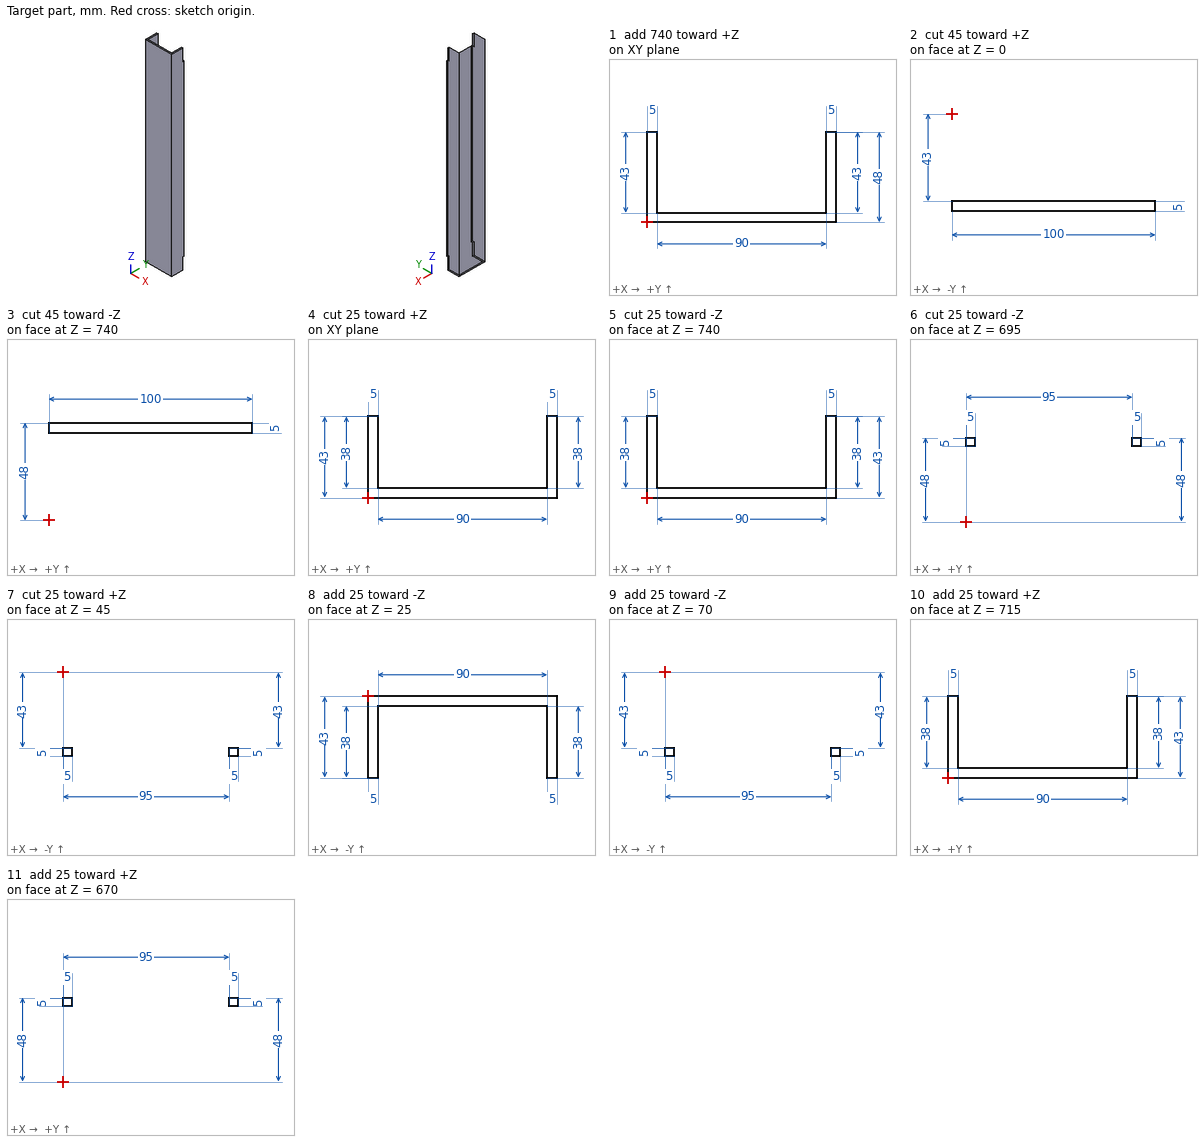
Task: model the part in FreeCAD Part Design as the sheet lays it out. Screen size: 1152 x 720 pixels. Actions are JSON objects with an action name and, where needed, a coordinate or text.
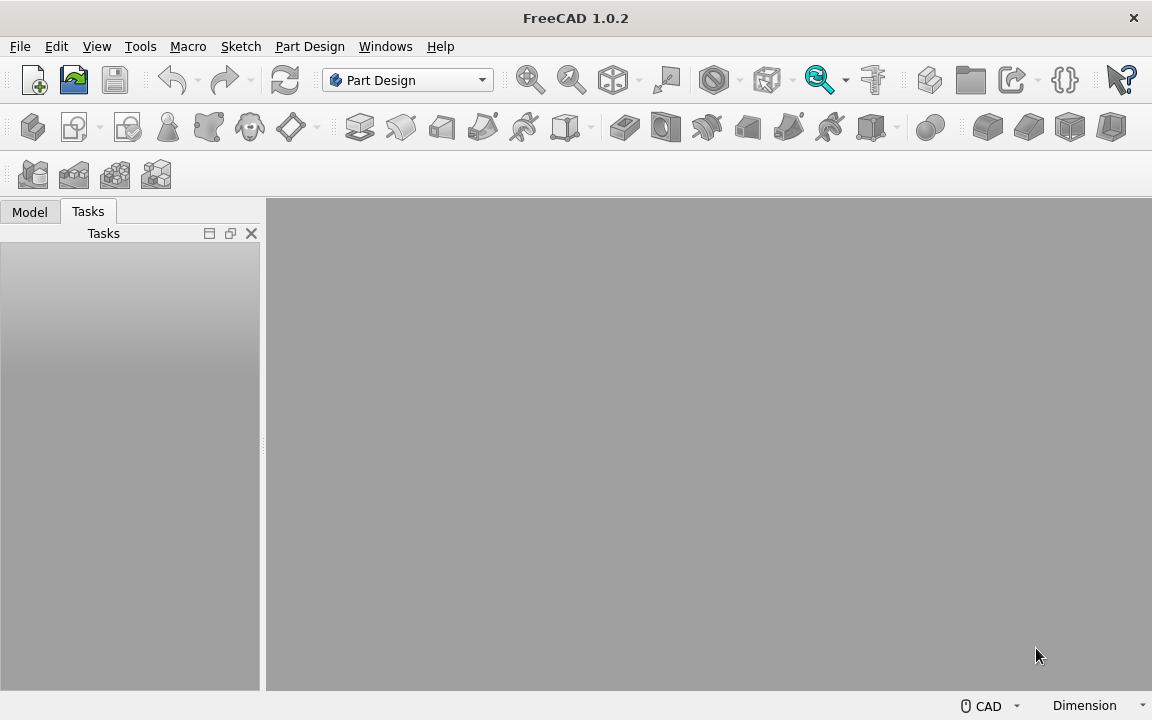
{"action": "left_click", "coordinate": [33, 80]}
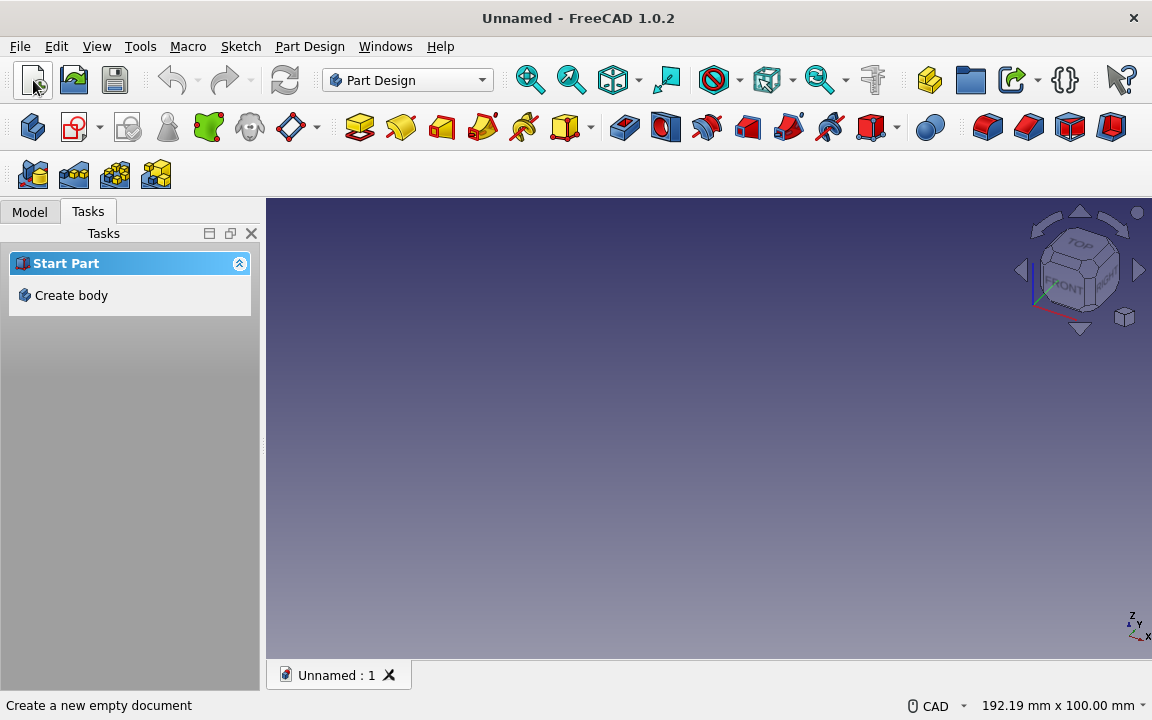
{"action": "left_click", "coordinate": [74, 128]}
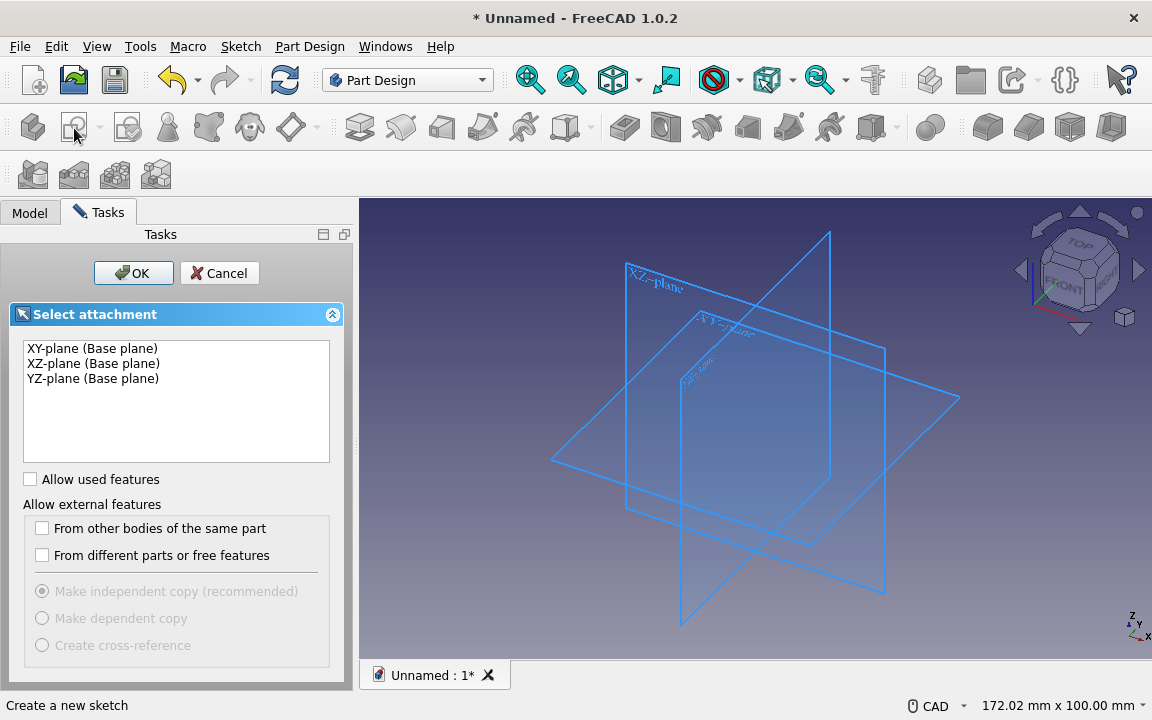
{"action": "left_click", "coordinate": [84, 348]}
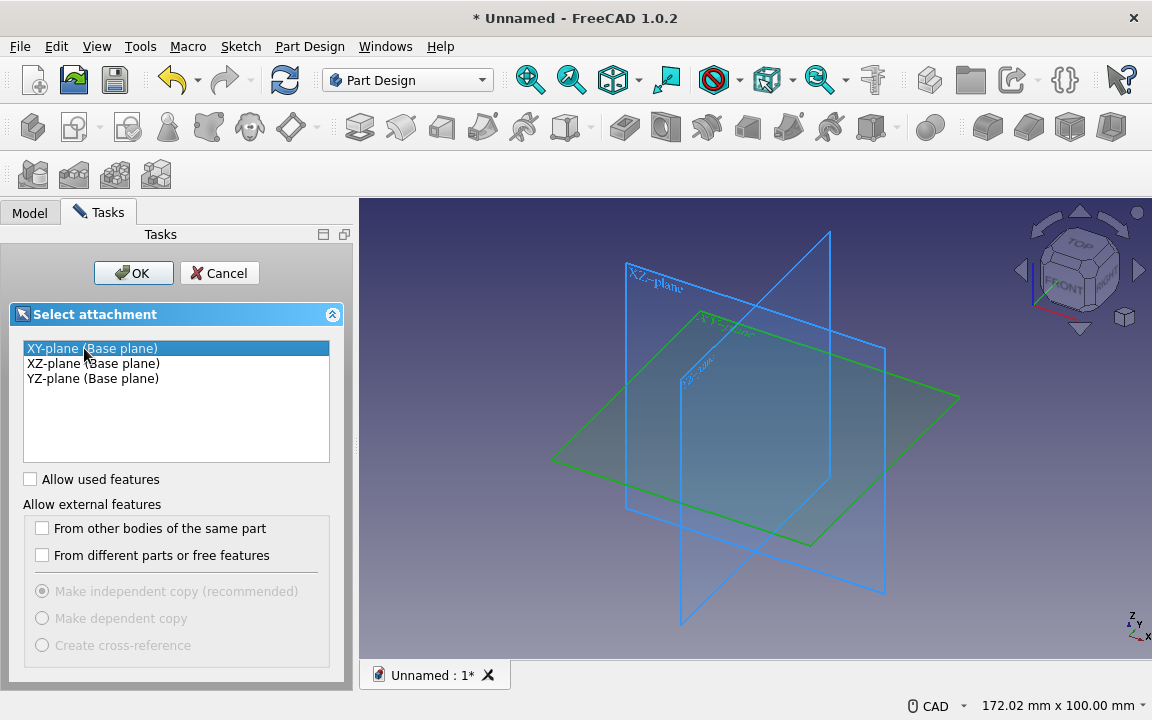
{"action": "left_click", "coordinate": [134, 273]}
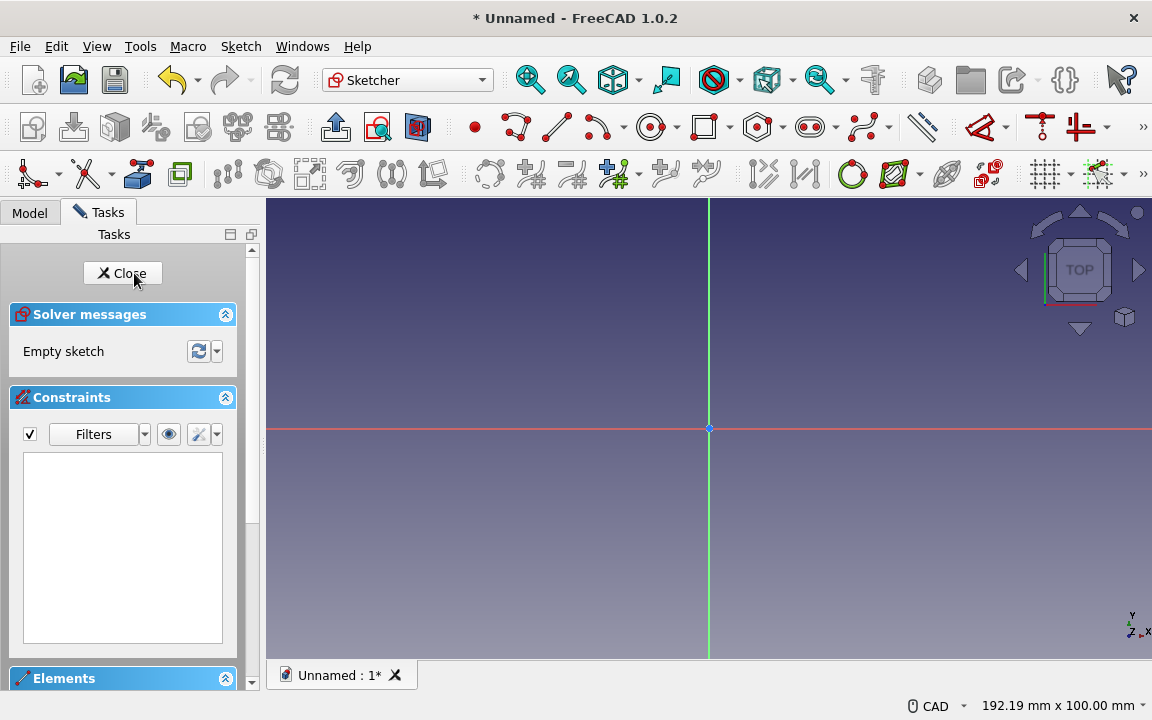
{"action": "scroll", "coordinate": [294, 631], "scroll_direction": "down", "scroll_amount": 2}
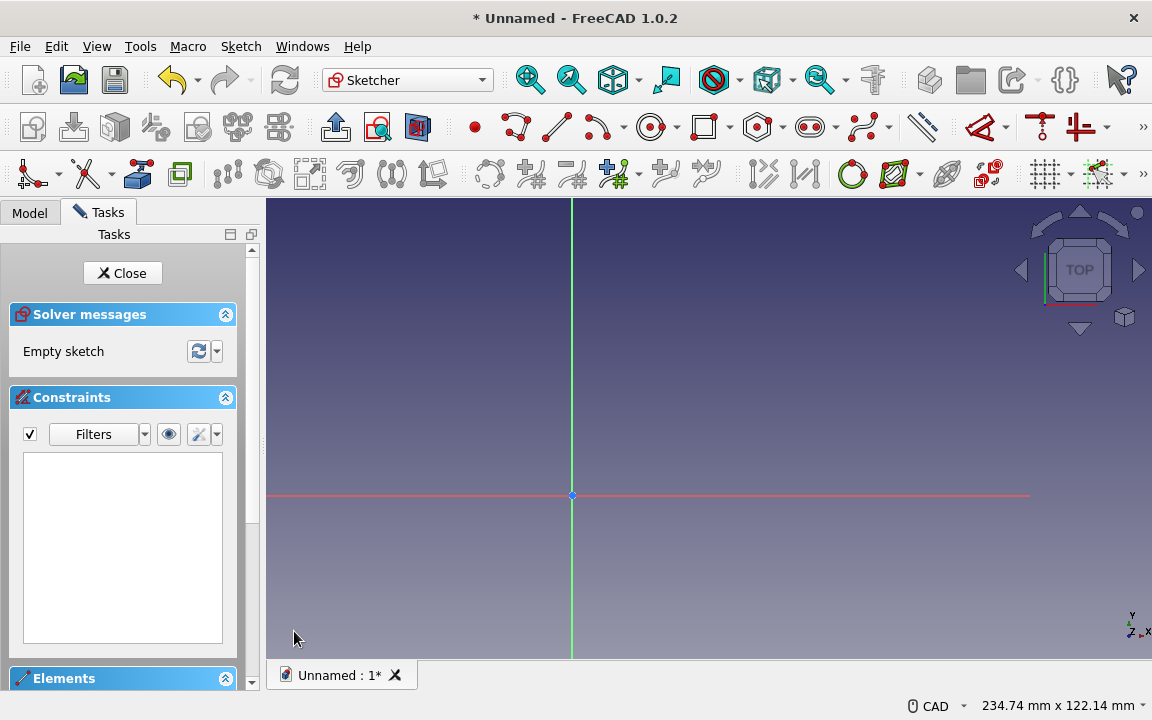
{"action": "scroll", "coordinate": [902, 407], "scroll_direction": "up", "scroll_amount": 2}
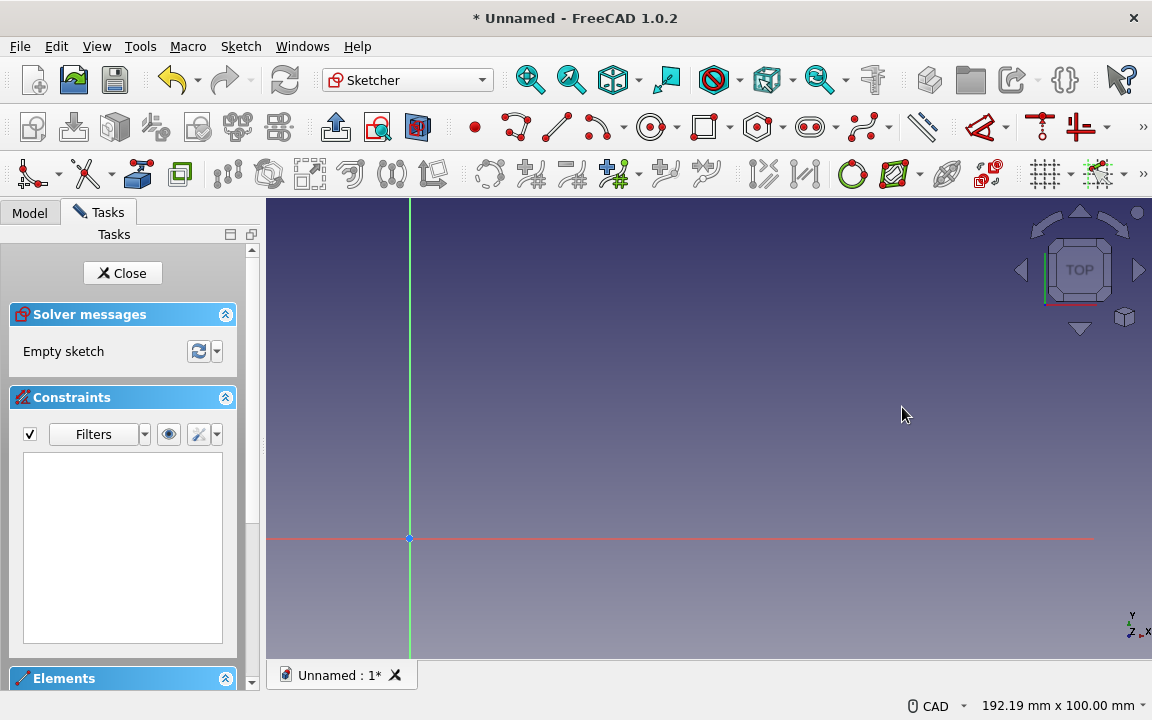
{"action": "left_click", "coordinate": [516, 128]}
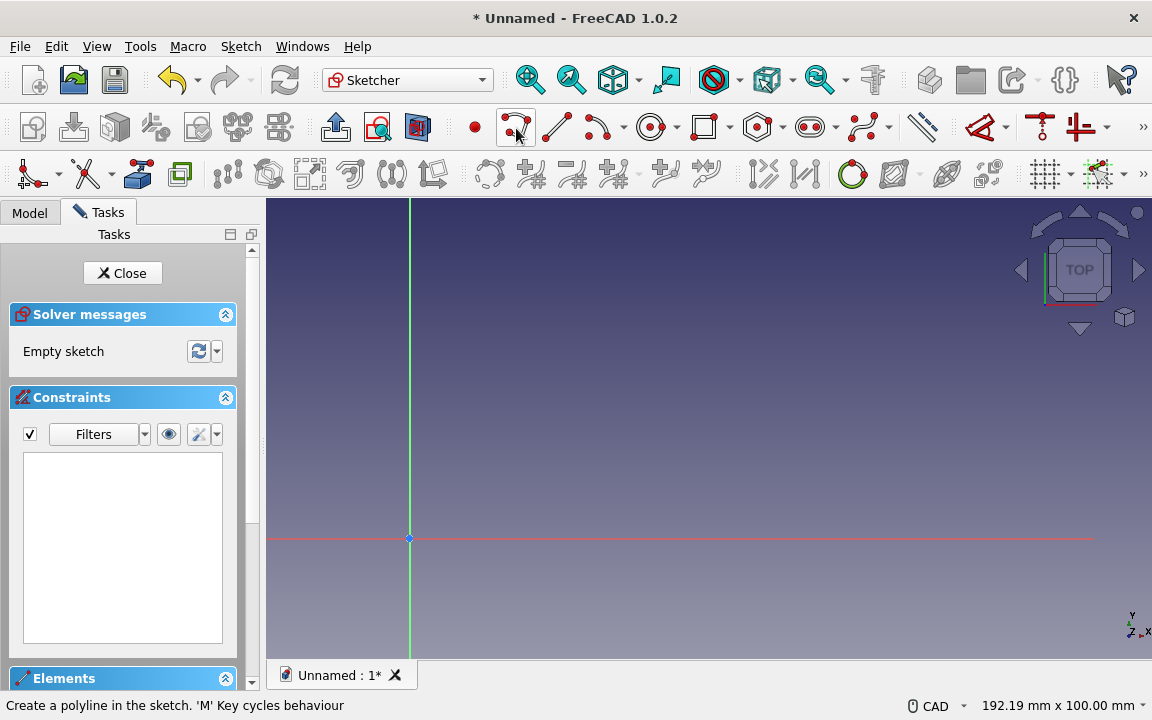
{"action": "left_click", "coordinate": [410, 539]}
{"action": "left_click", "coordinate": [871, 530]}
{"action": "left_click", "coordinate": [871, 318]}
{"action": "left_click", "coordinate": [848, 318]}
{"action": "left_click", "coordinate": [848, 516]}
{"action": "left_click", "coordinate": [433, 516]}
{"action": "left_click", "coordinate": [433, 318]}
{"action": "left_click", "coordinate": [419, 318]}
{"action": "left_click", "coordinate": [410, 539]}
{"action": "key", "text": "Escape"}
{"action": "key", "text": "Escape"}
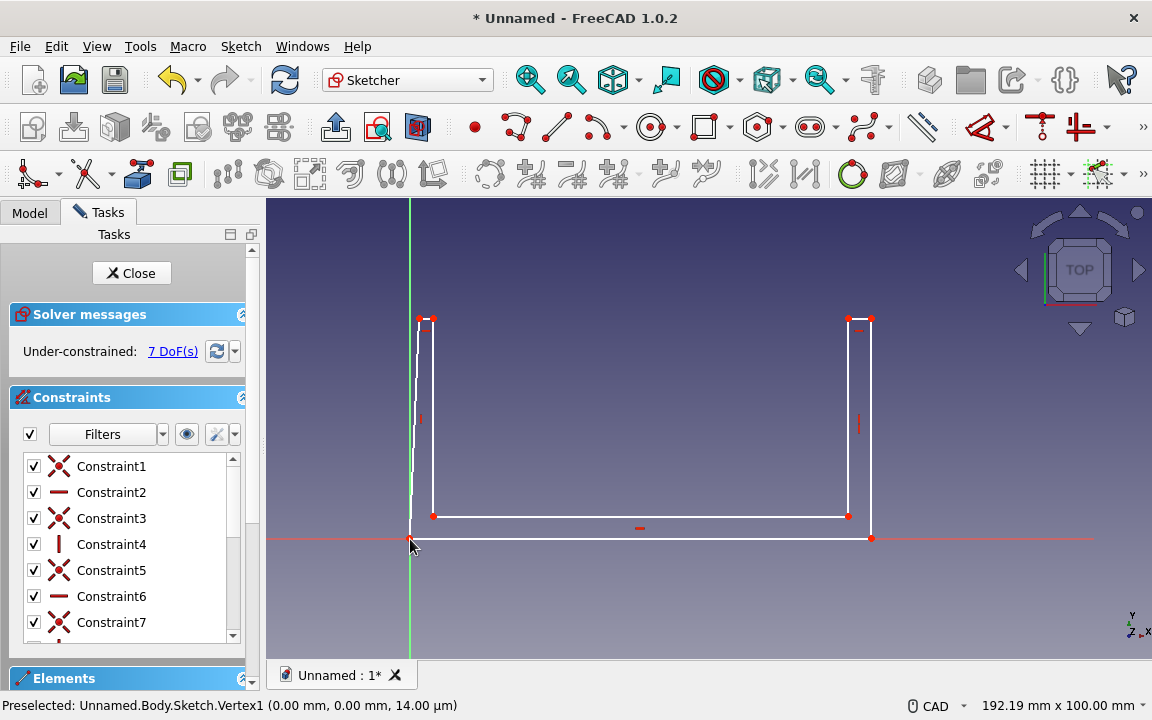
{"action": "left_click", "coordinate": [412, 473]}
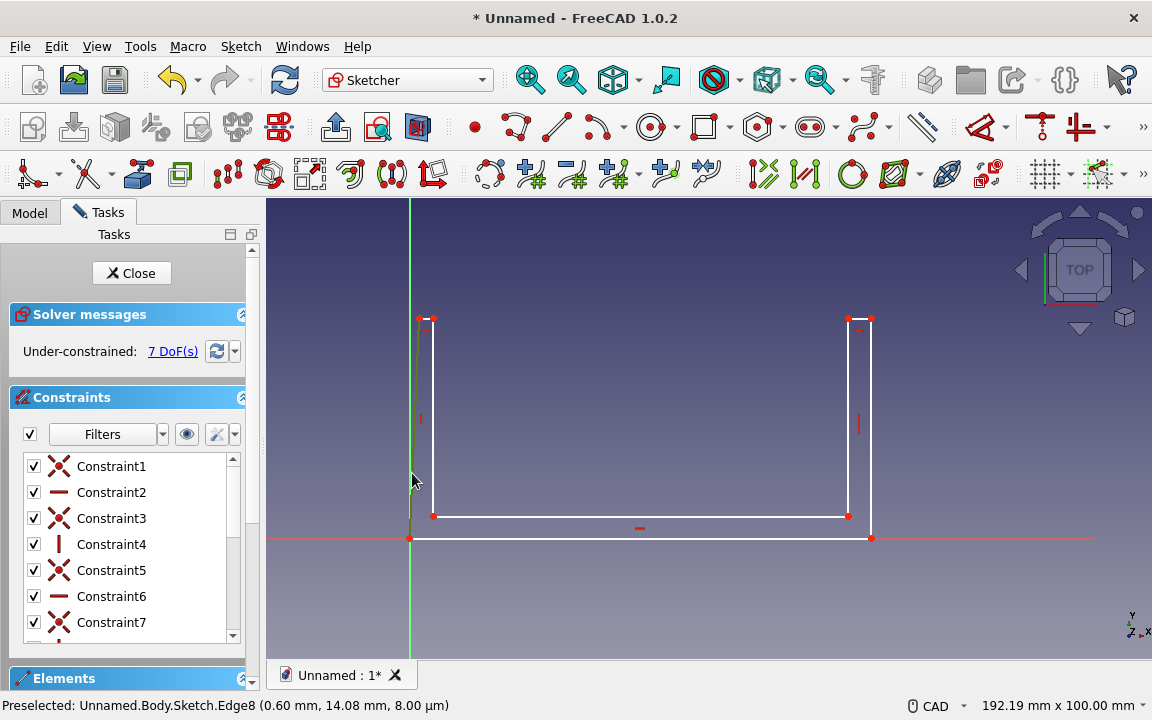
{"action": "key", "text": "v"}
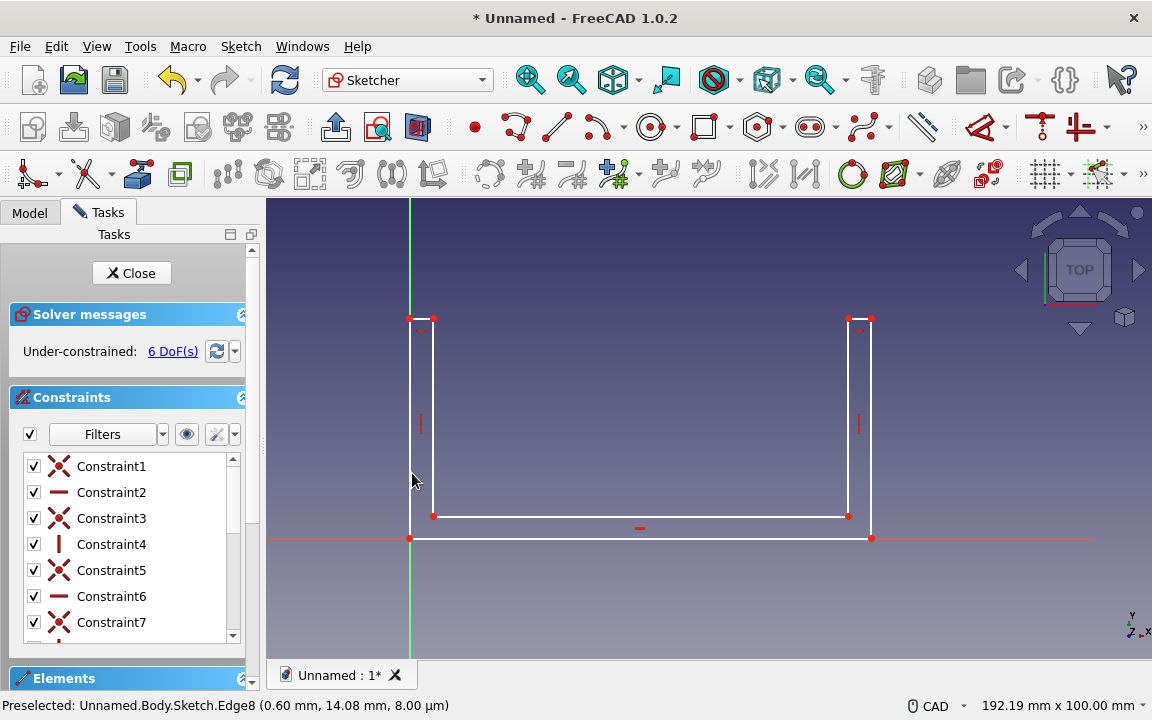
{"action": "scroll", "coordinate": [862, 319], "scroll_direction": "up", "scroll_amount": 3}